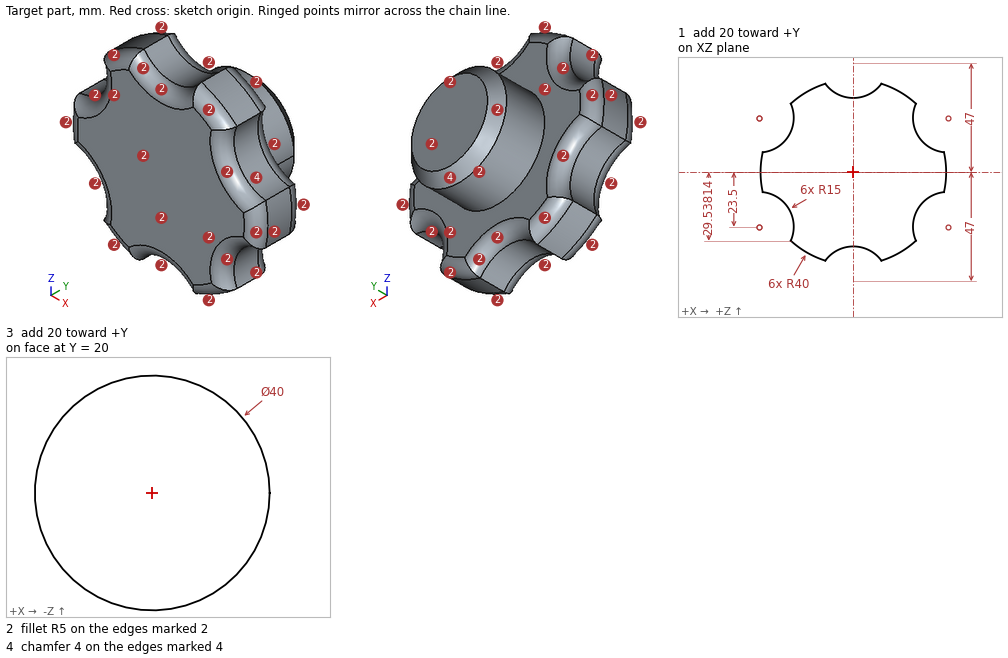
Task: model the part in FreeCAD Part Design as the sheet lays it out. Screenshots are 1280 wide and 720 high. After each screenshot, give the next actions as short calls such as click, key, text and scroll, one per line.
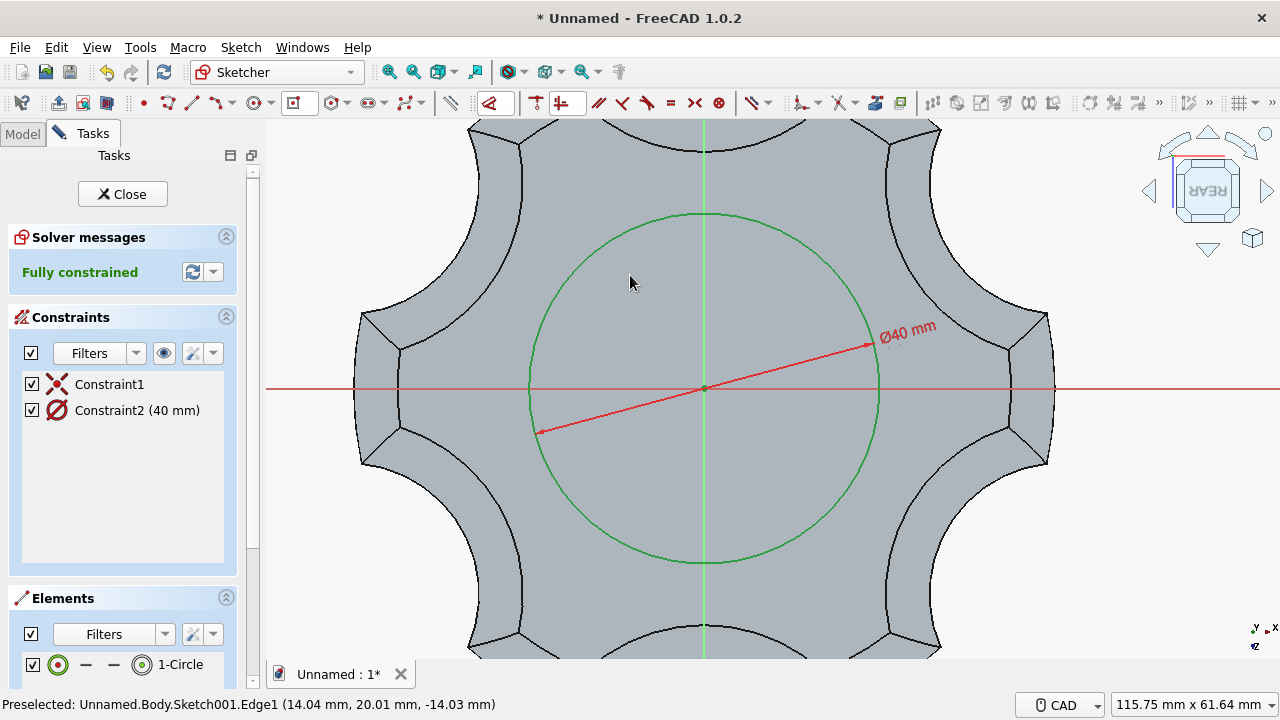
click(123, 194)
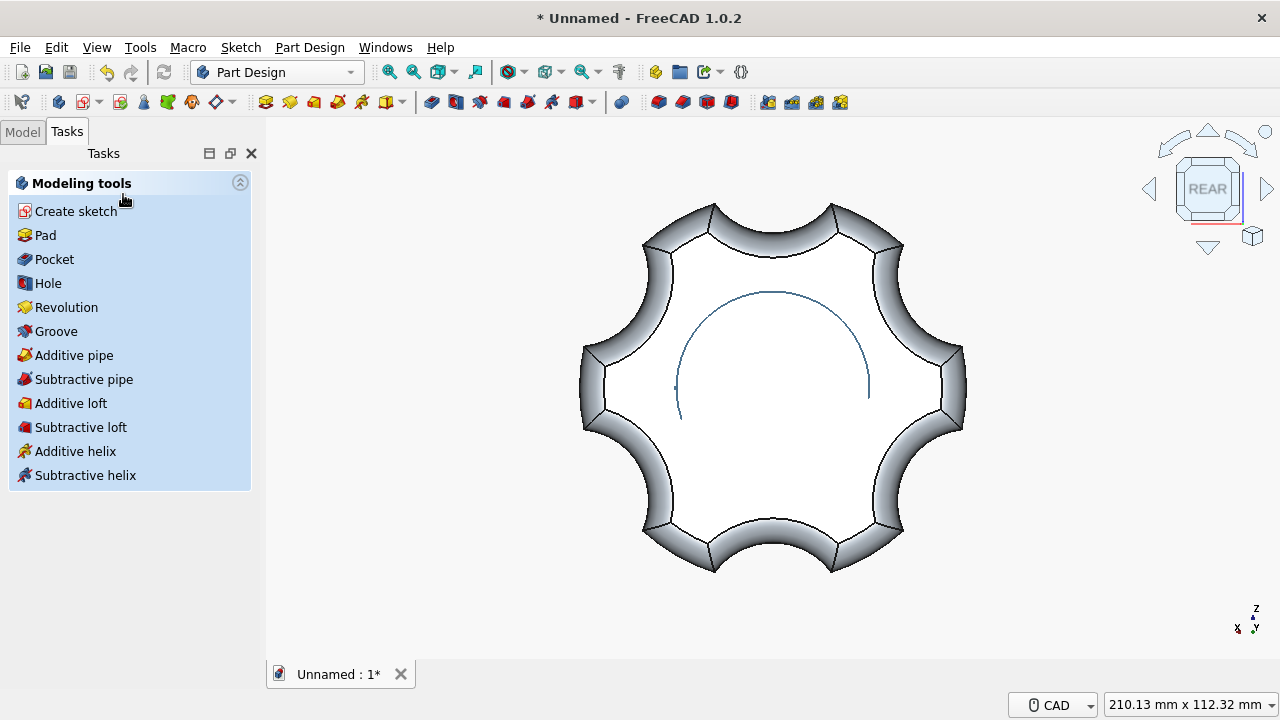
click(266, 102)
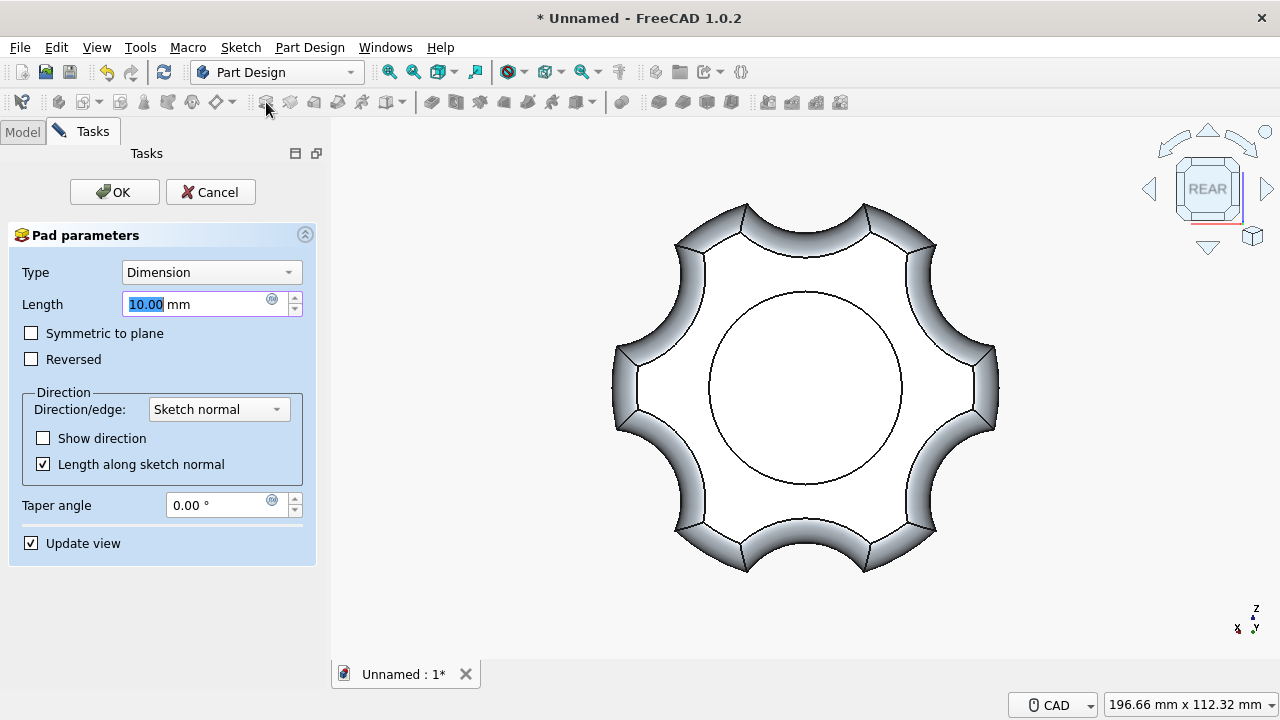
text(20)
key(Tab)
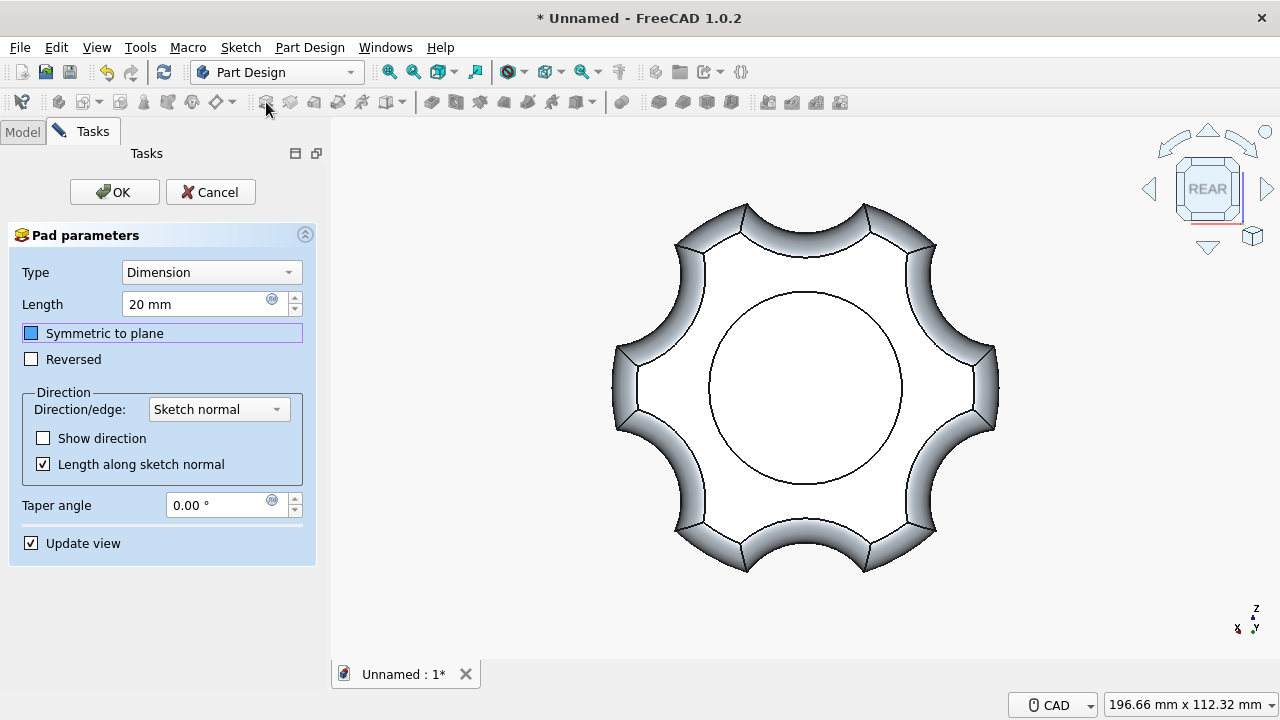
click(115, 192)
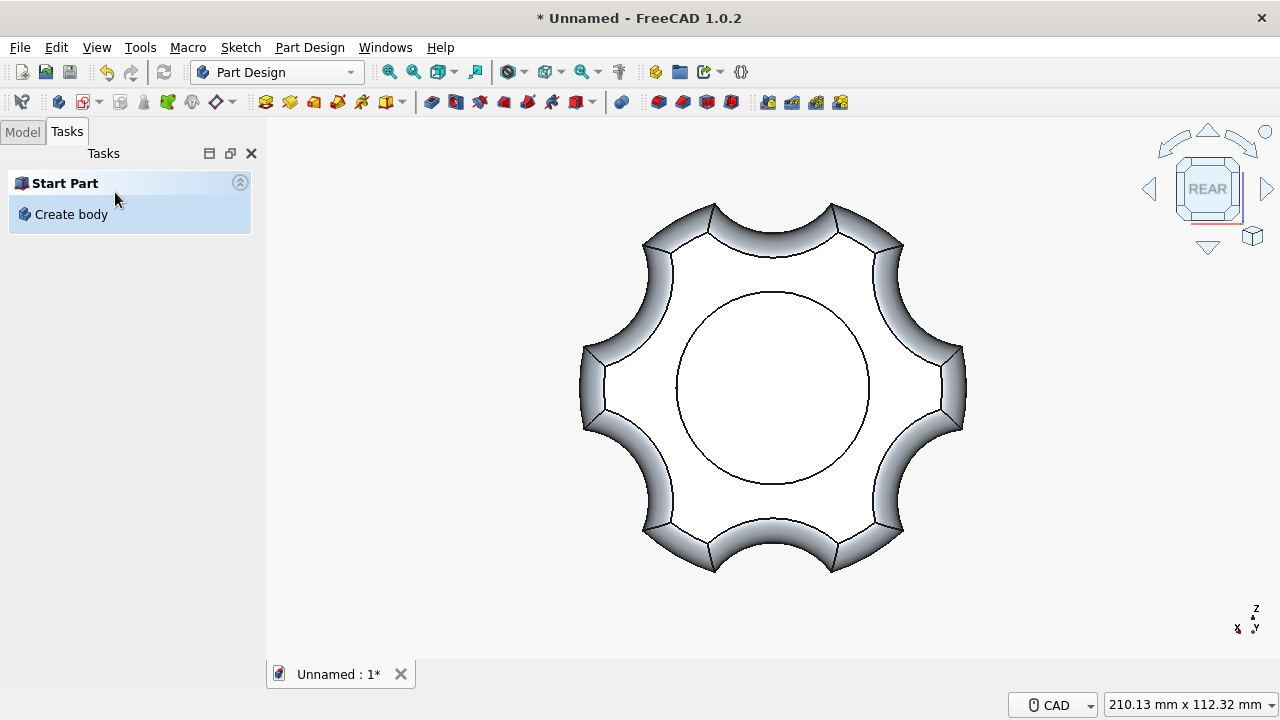
click(870, 387)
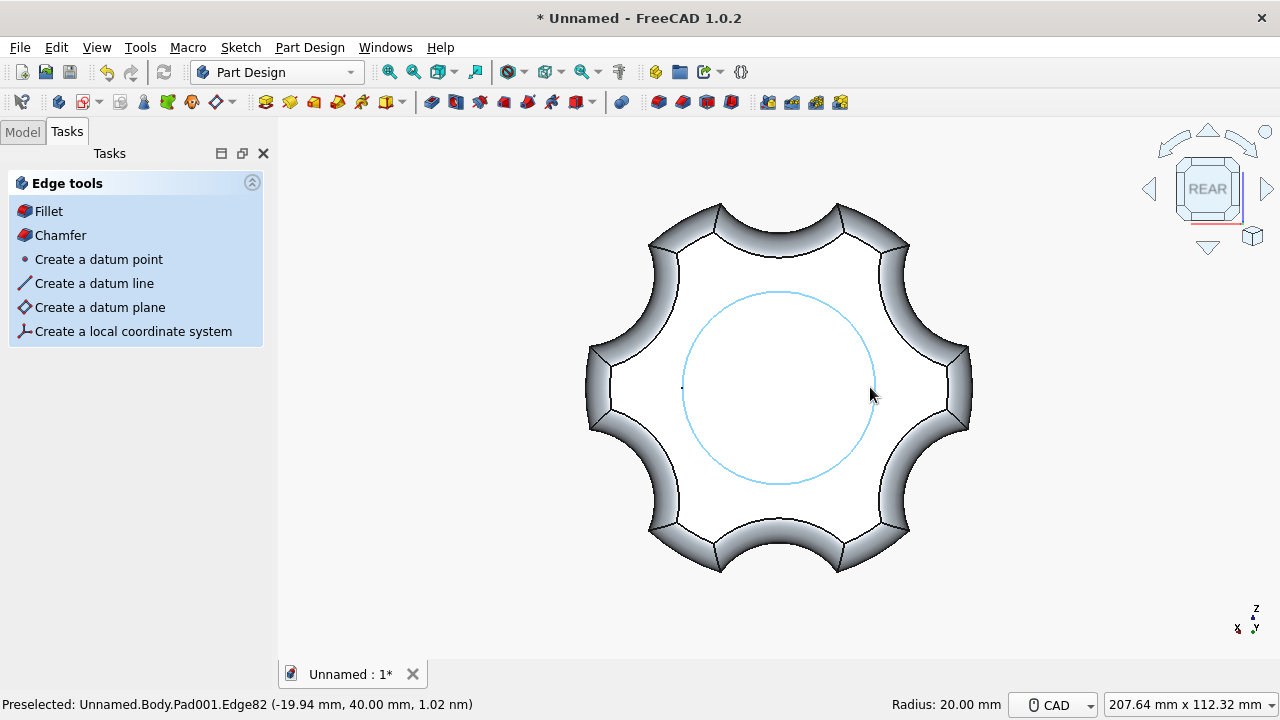
click(684, 102)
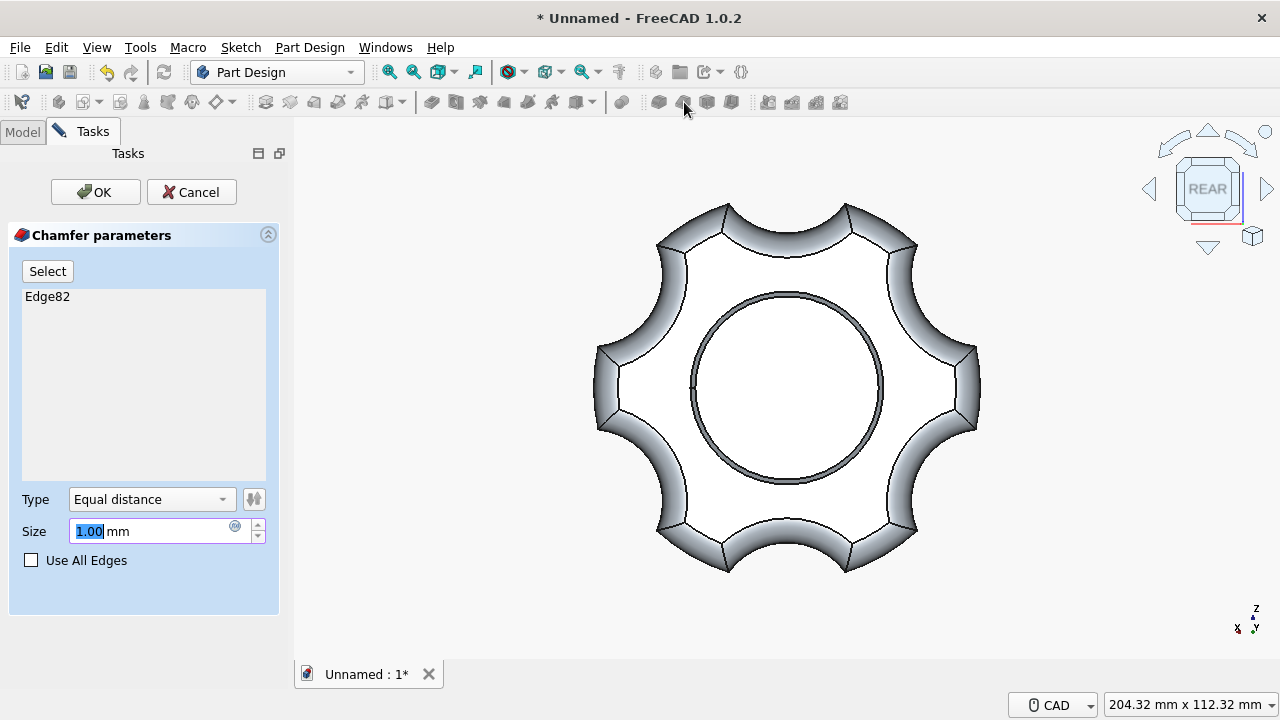
text(4)
key(Tab)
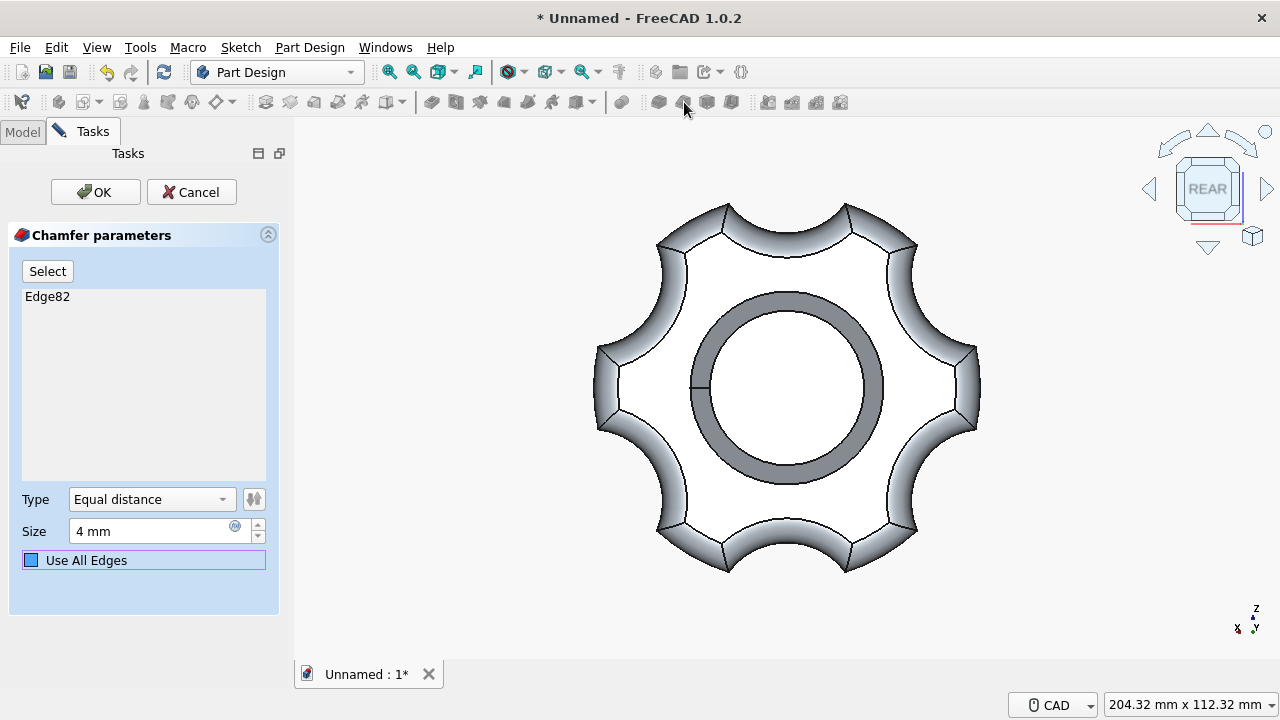
click(96, 192)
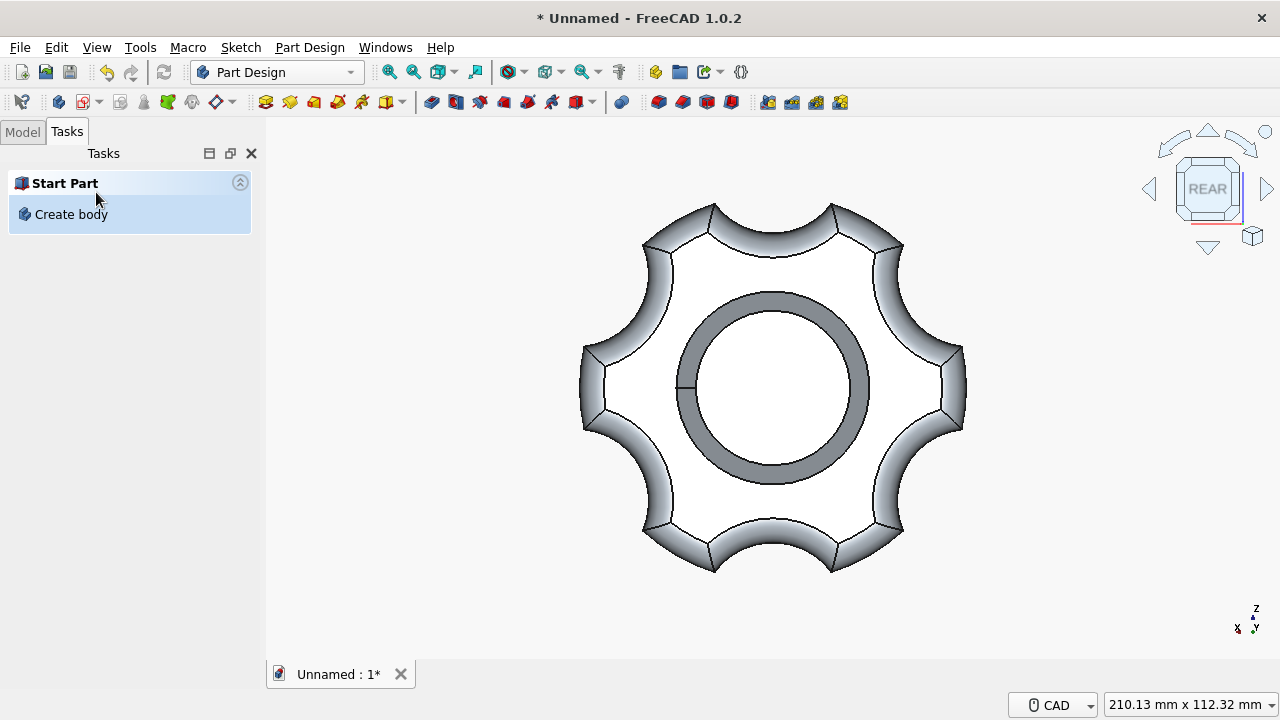
key(0)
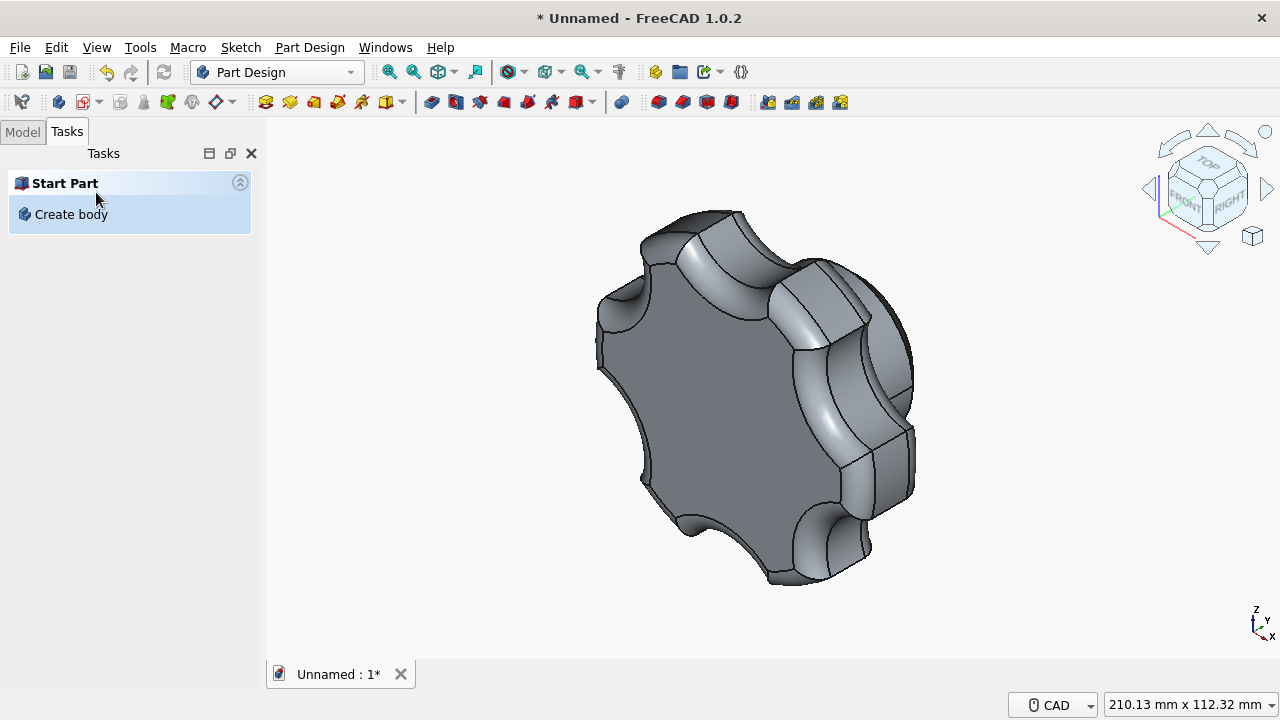
click(390, 72)